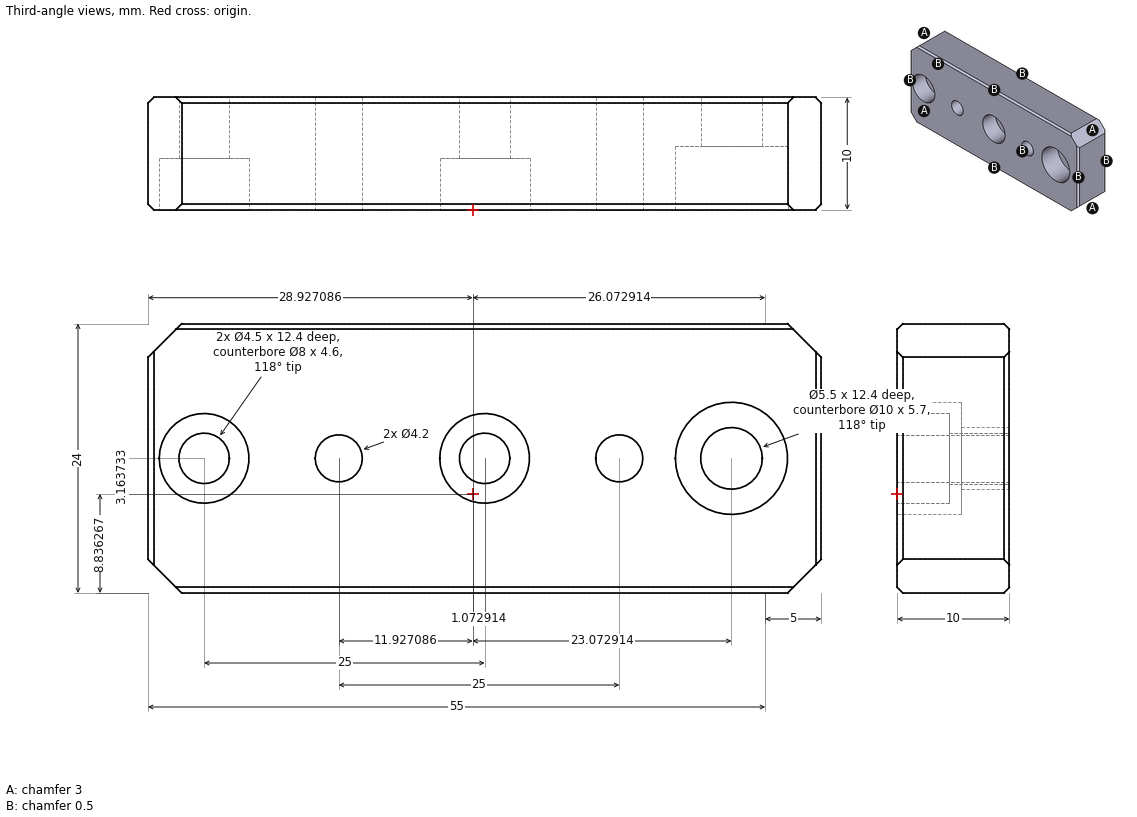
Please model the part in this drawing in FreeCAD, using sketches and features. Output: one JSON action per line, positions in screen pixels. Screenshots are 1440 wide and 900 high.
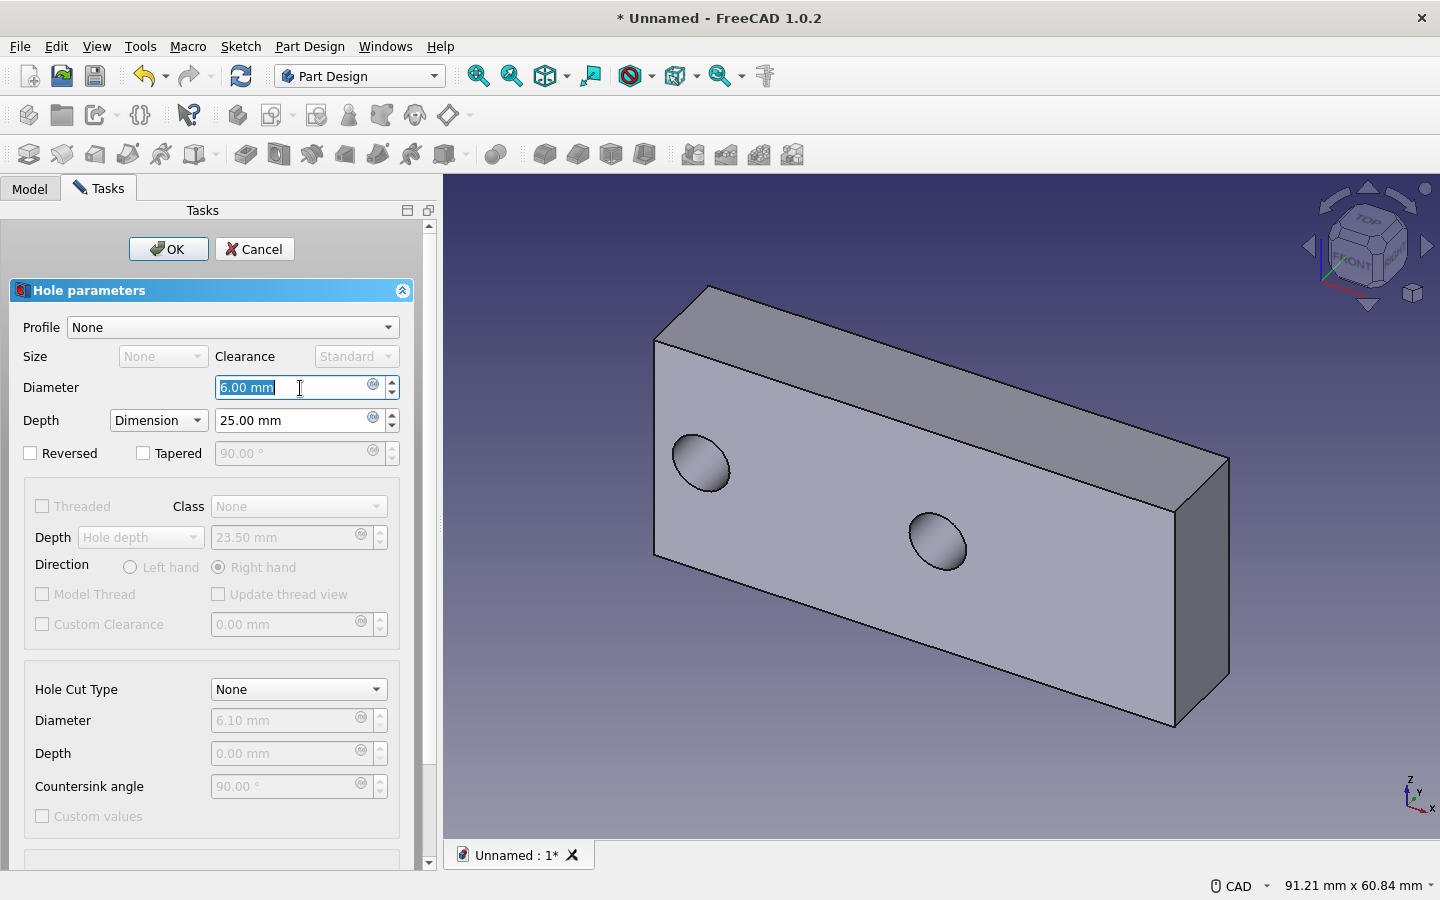
{"action": "type", "text": "4.5"}
{"action": "key", "text": "Tab"}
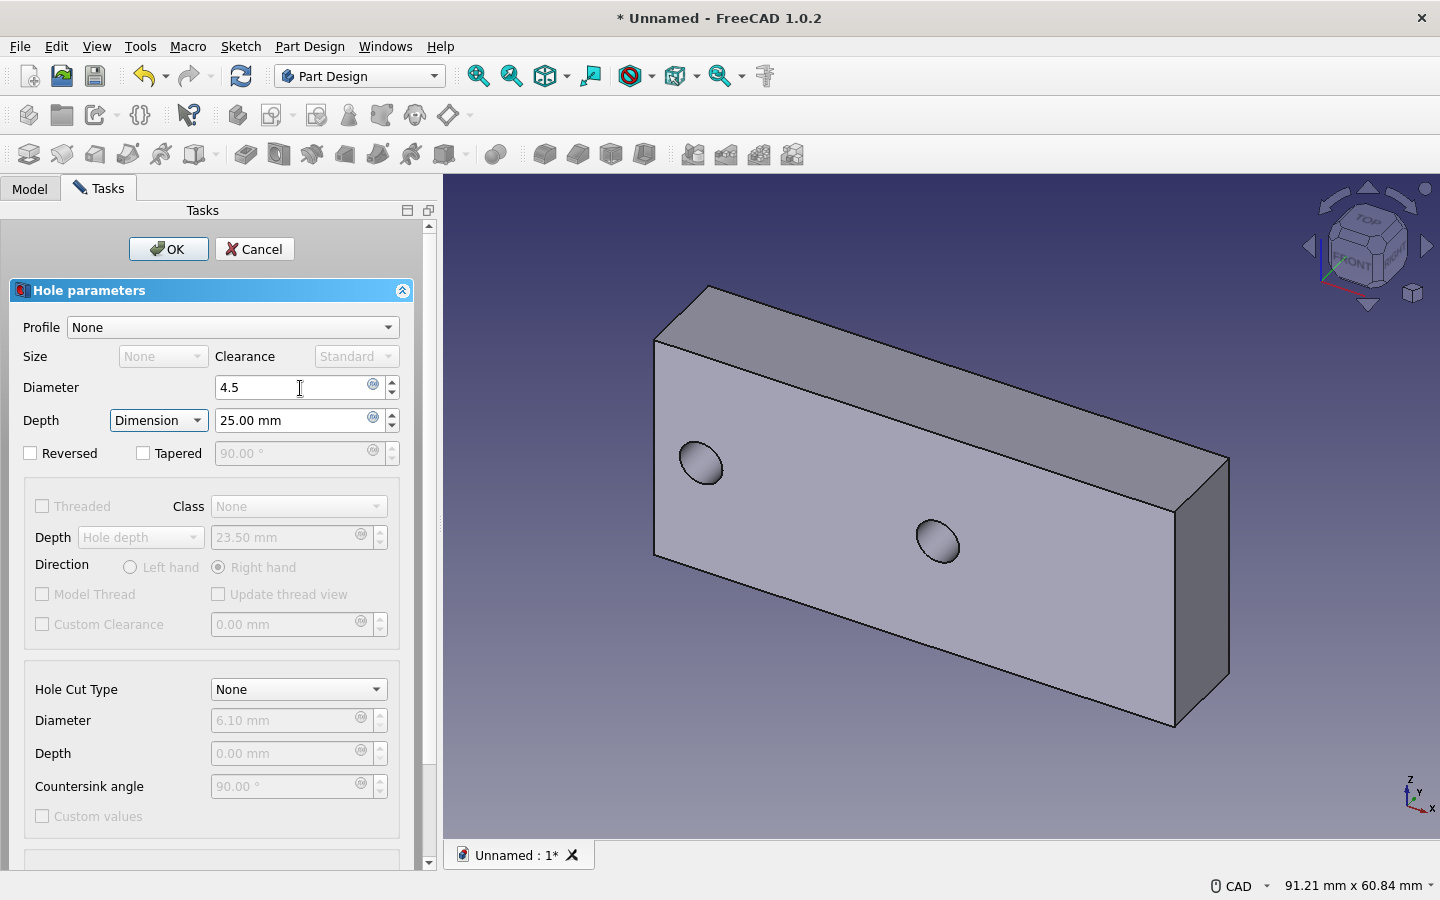
{"action": "triple_click", "coordinate": [300, 420]}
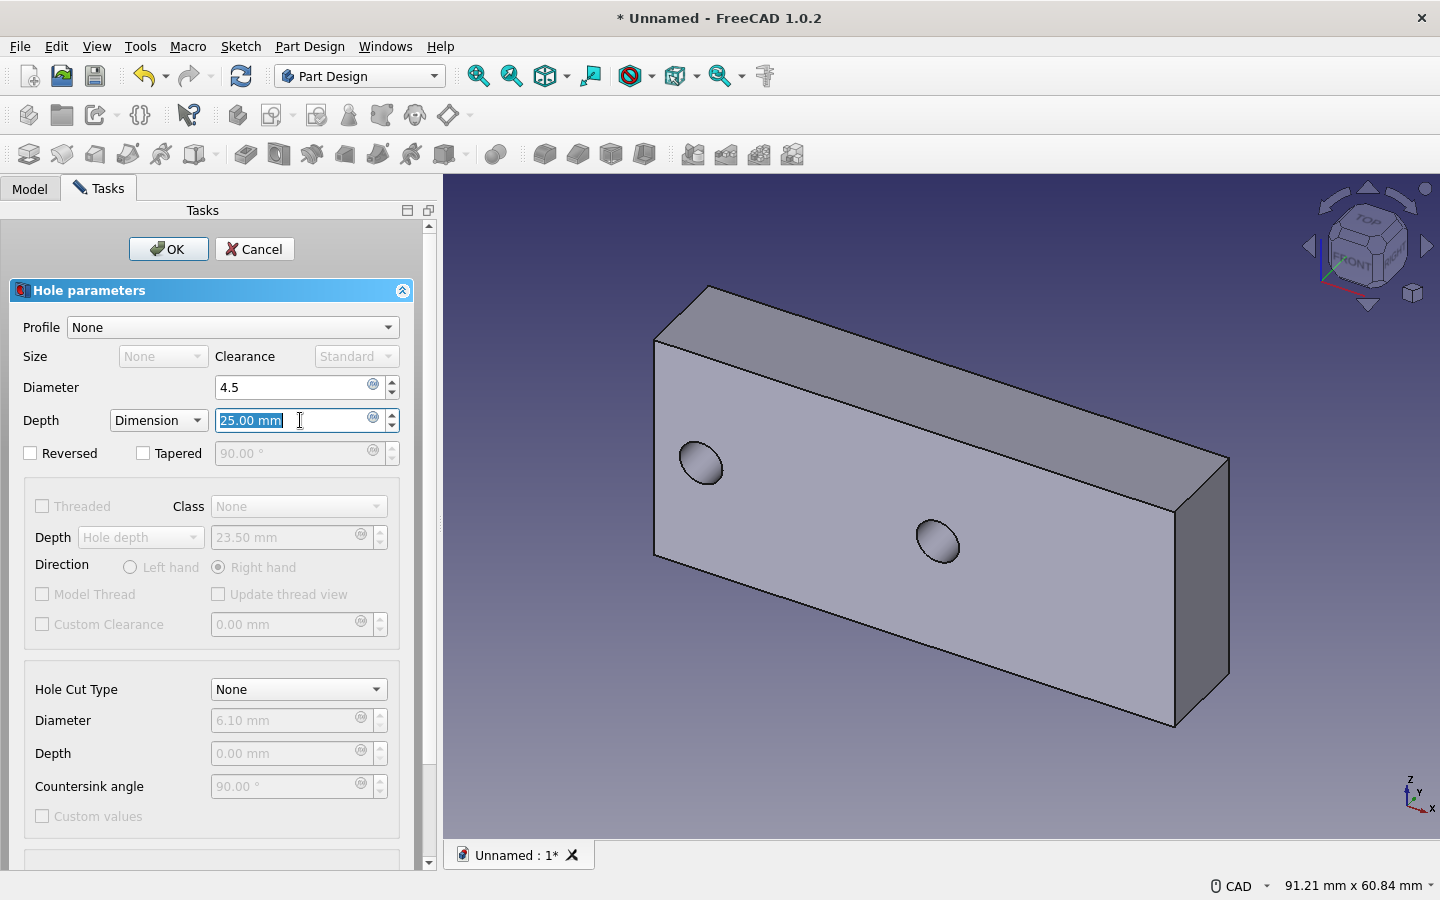
{"action": "type", "text": "12.4"}
{"action": "key", "text": "Tab"}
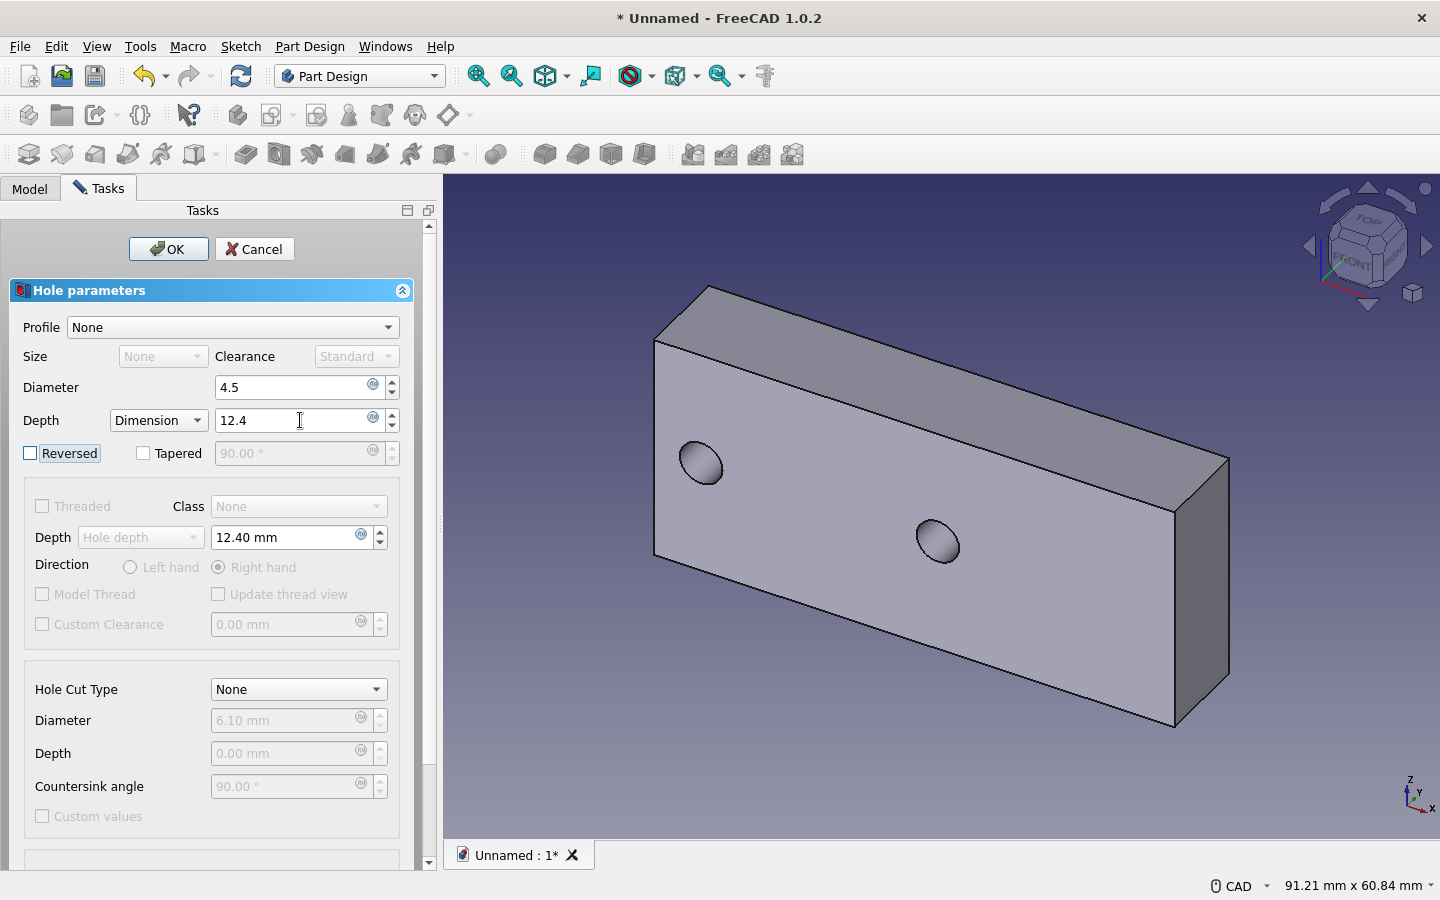
{"action": "left_click", "coordinate": [300, 690]}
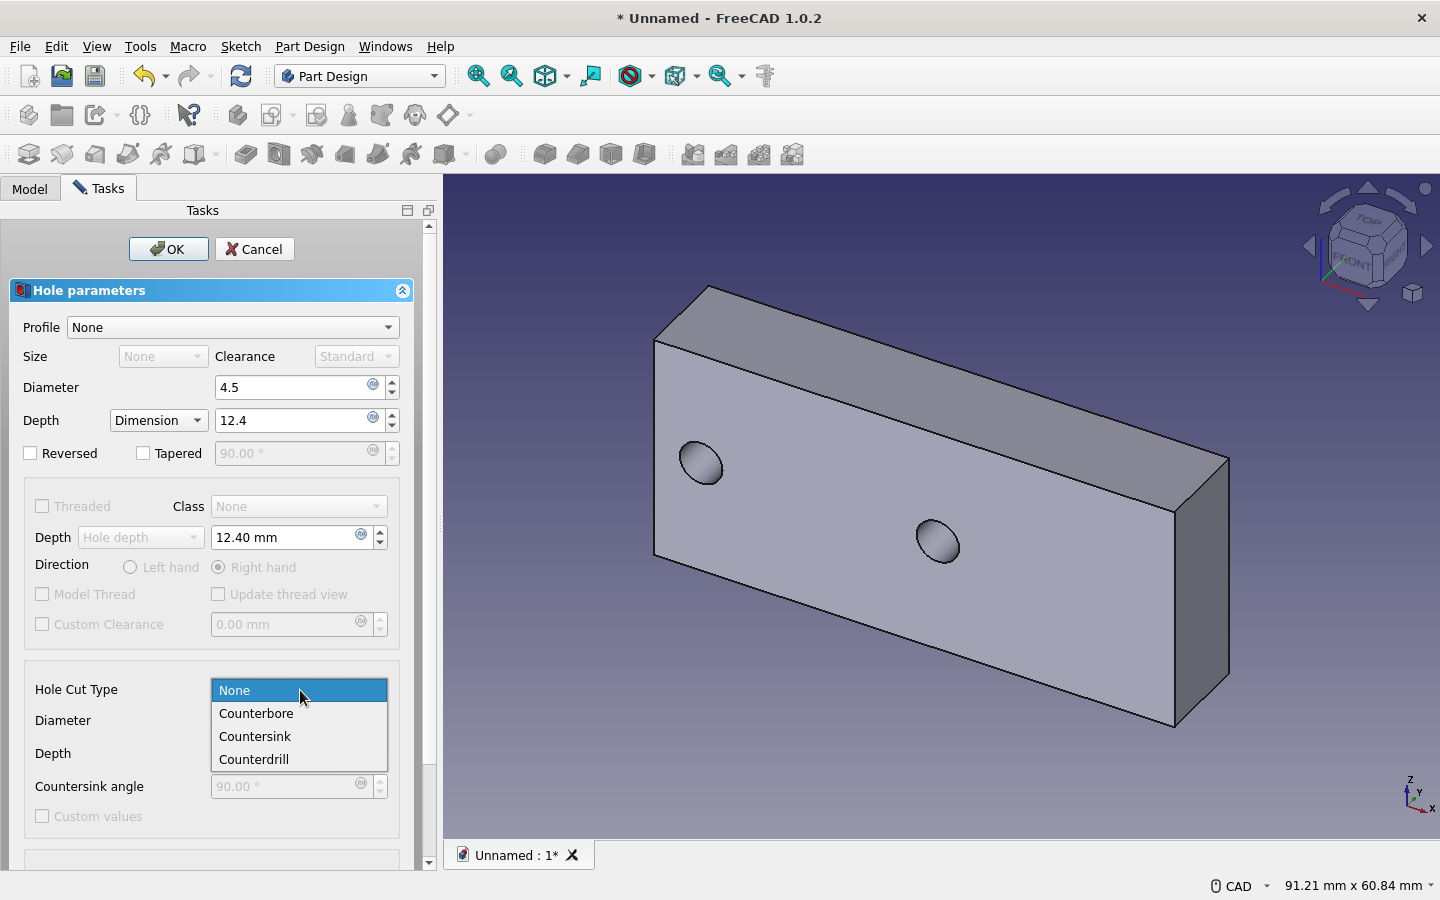
{"action": "left_click", "coordinate": [298, 714]}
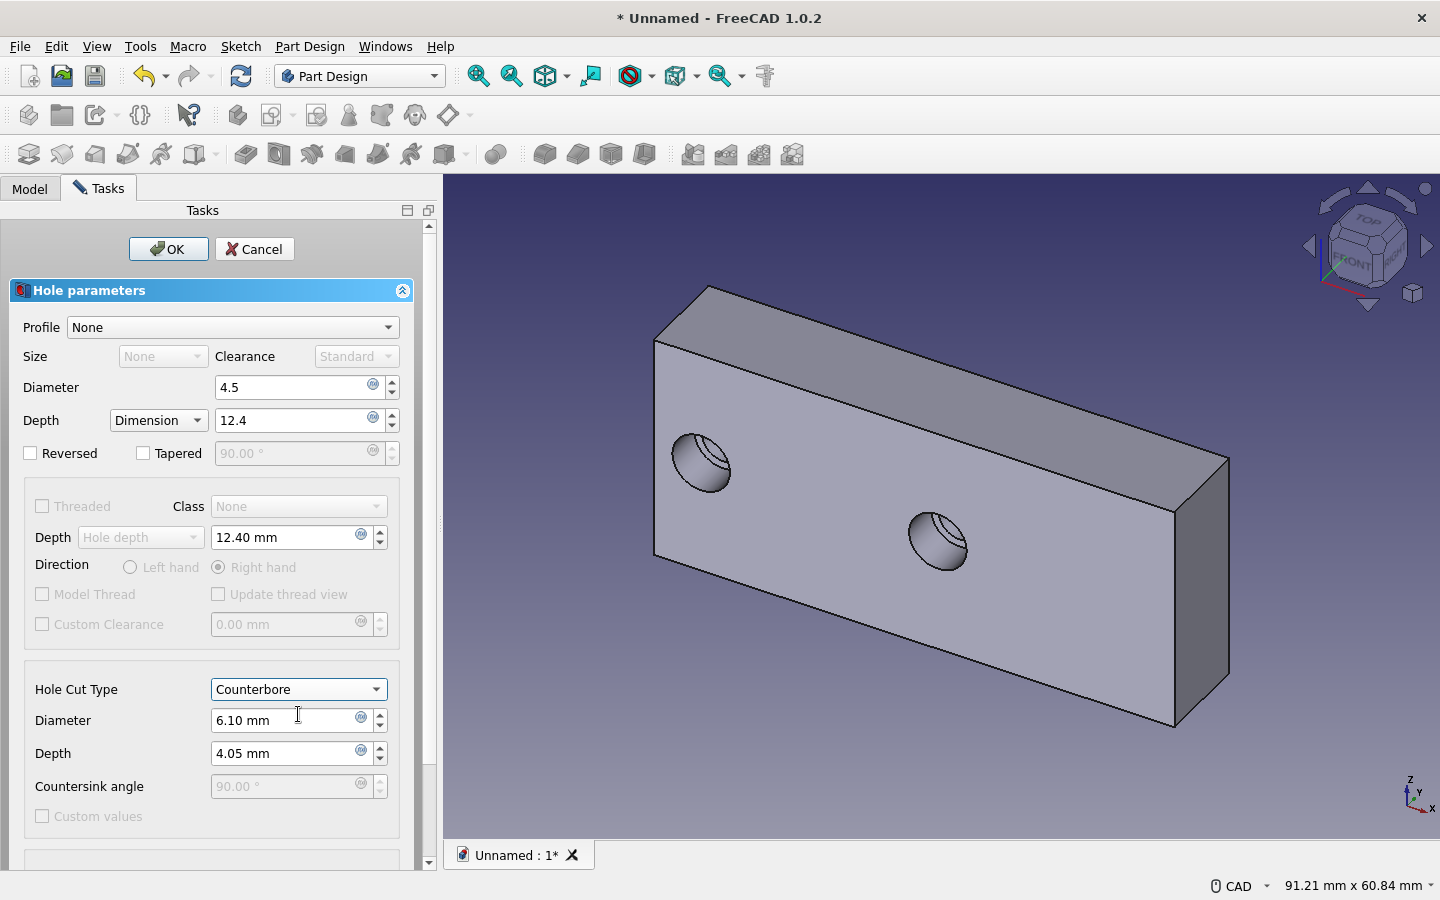
{"action": "triple_click", "coordinate": [292, 720]}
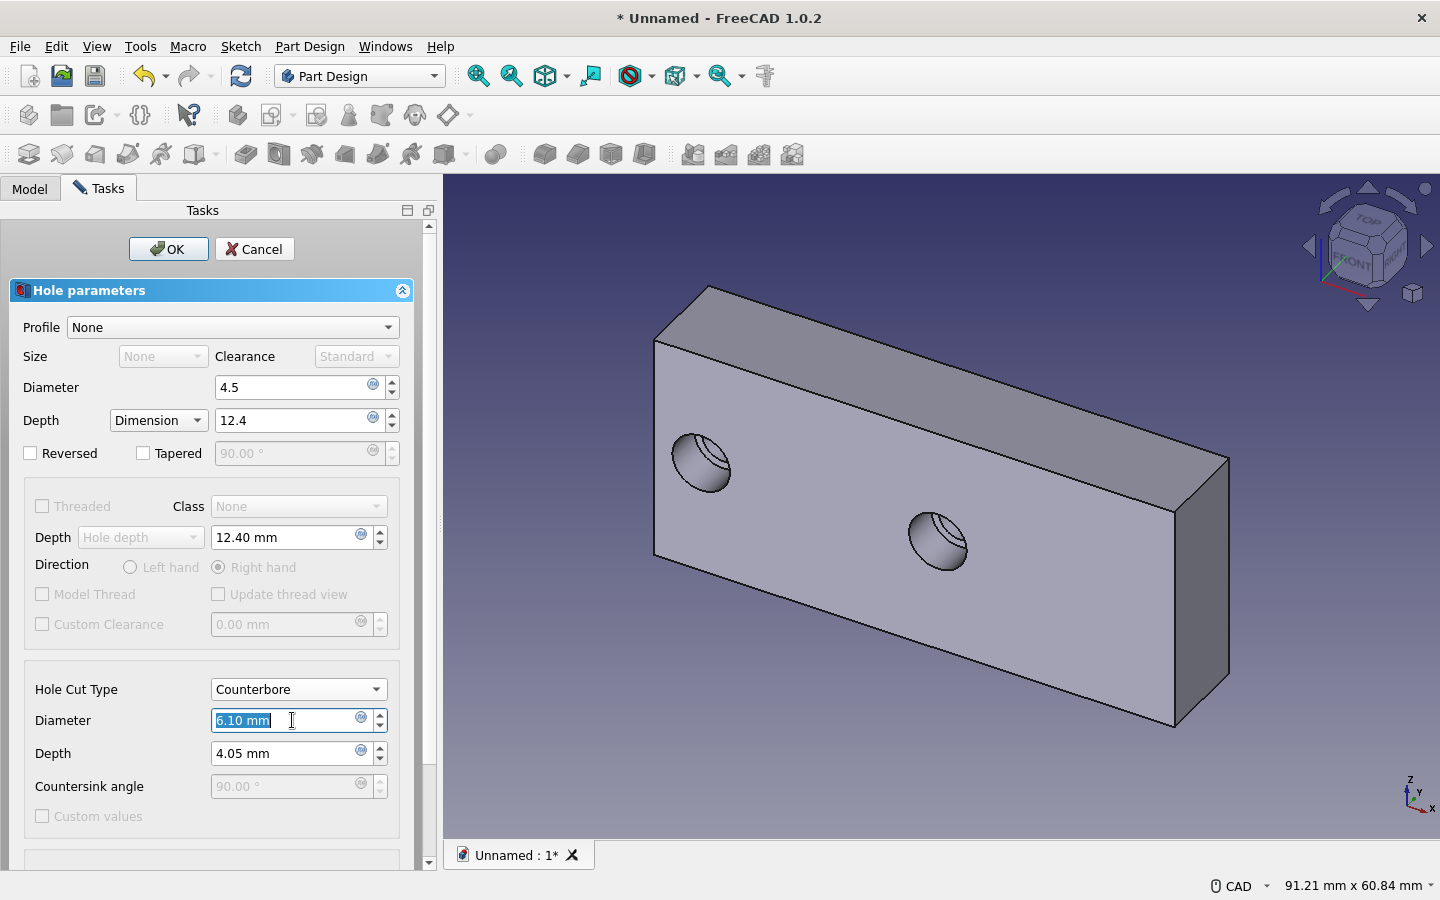
{"action": "type", "text": "8"}
{"action": "key", "text": "Tab"}